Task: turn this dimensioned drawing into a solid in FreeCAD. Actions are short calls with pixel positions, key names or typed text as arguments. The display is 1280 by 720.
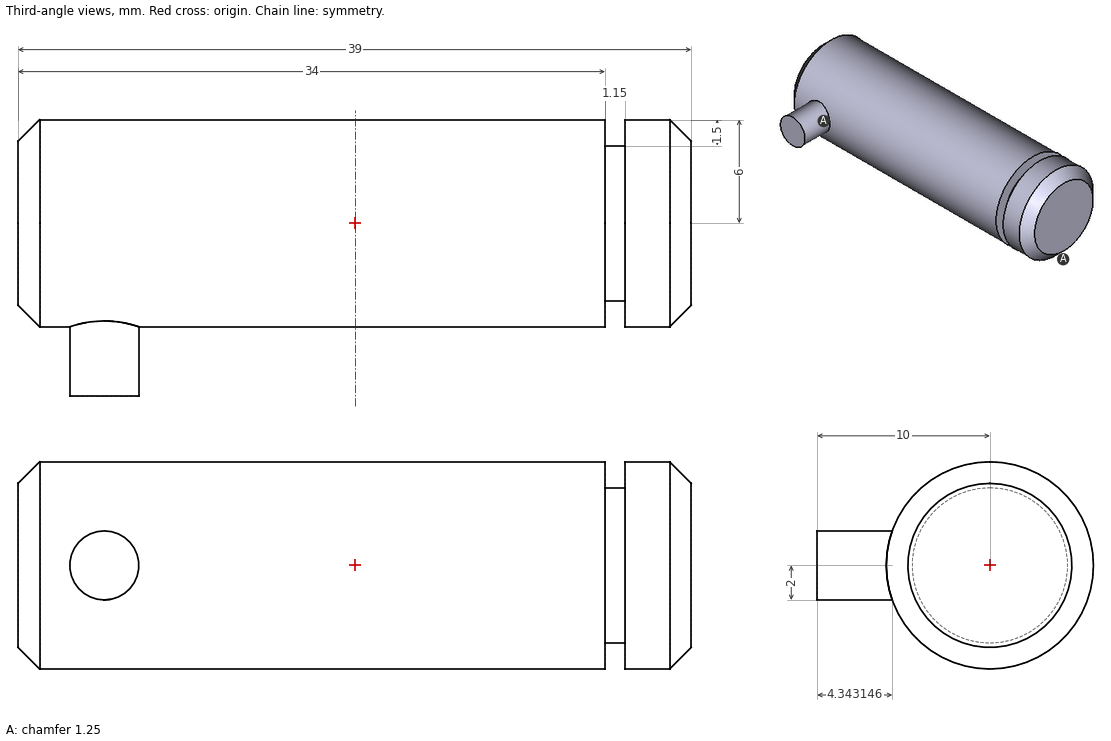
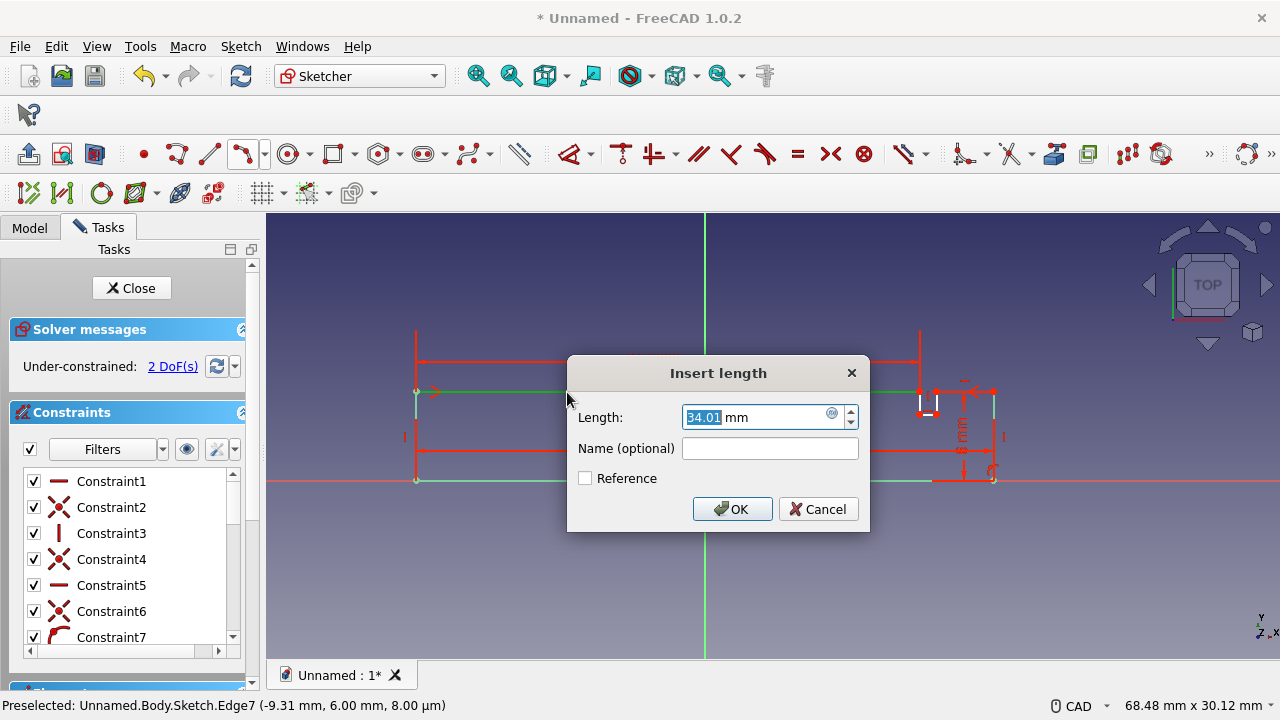
text(34)
key(Return)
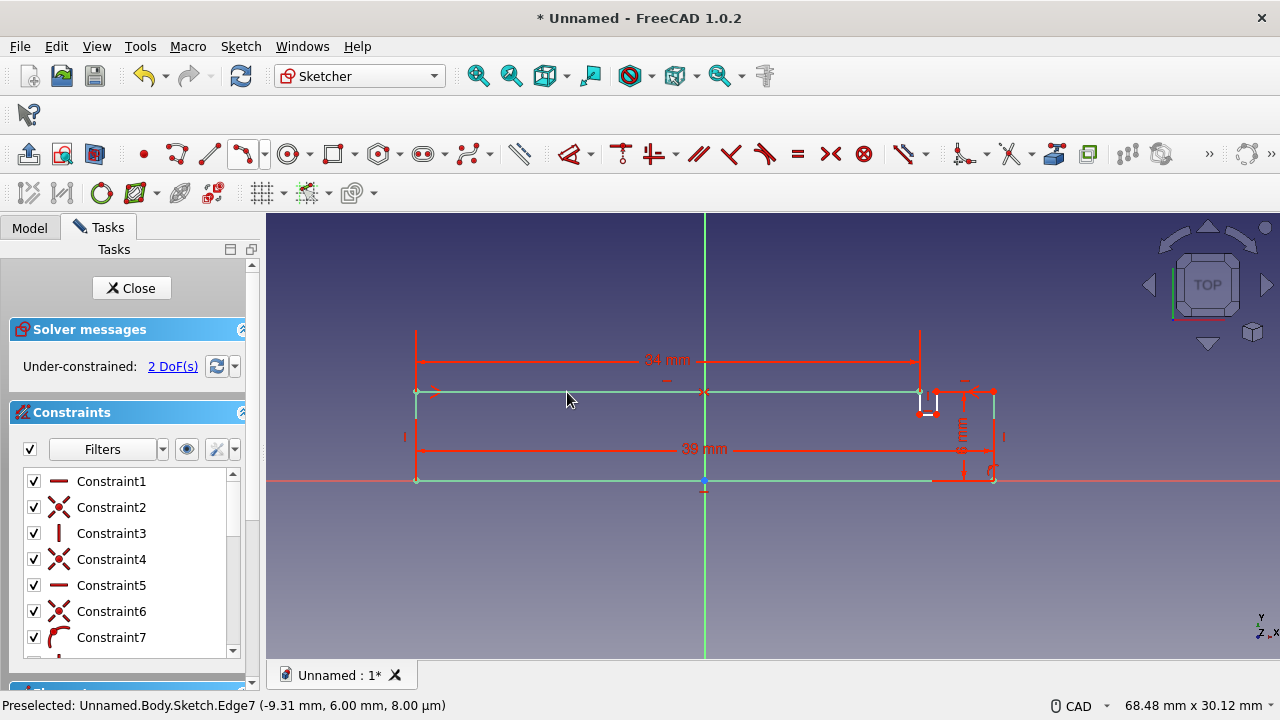
scroll(937, 406, up, 3)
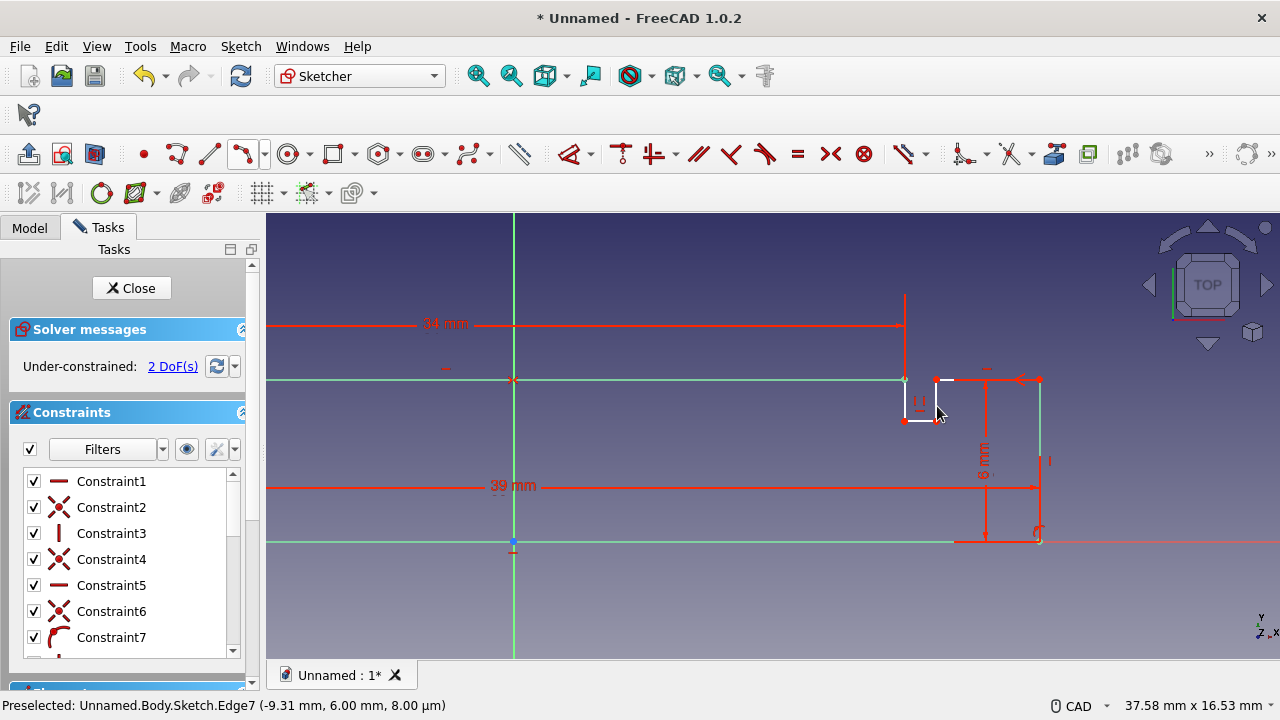
click(936, 405)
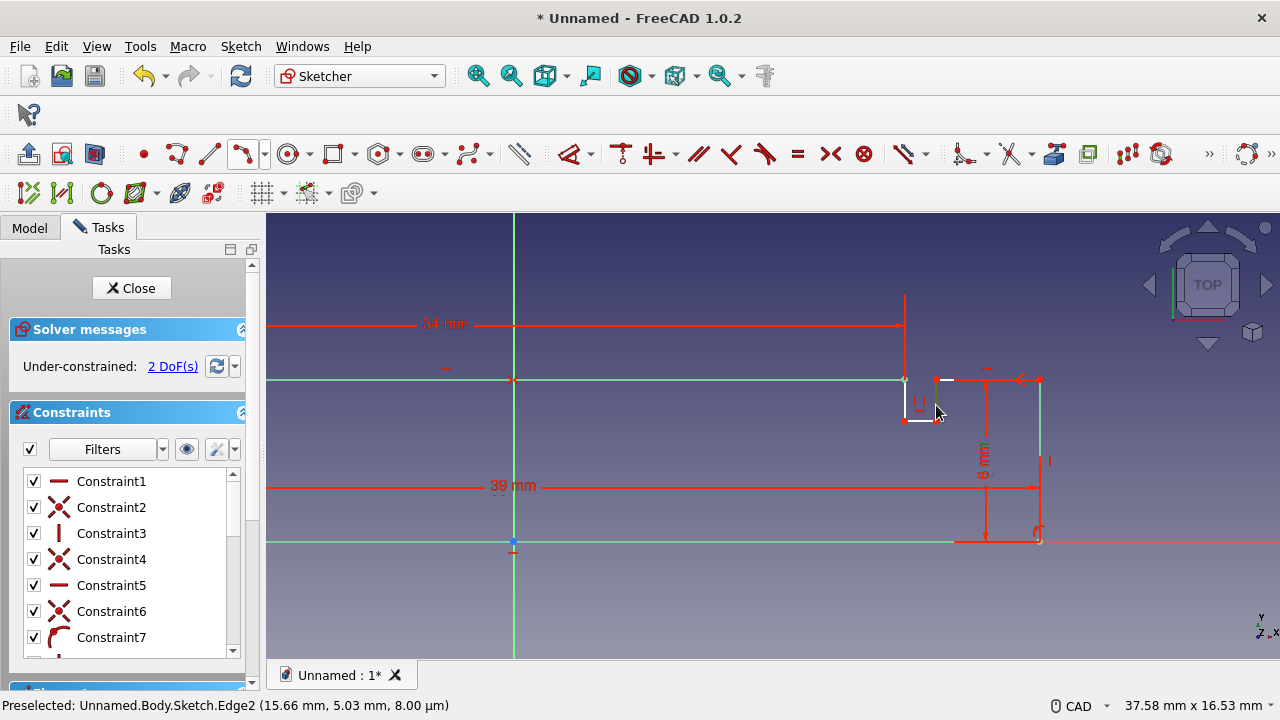
key(i)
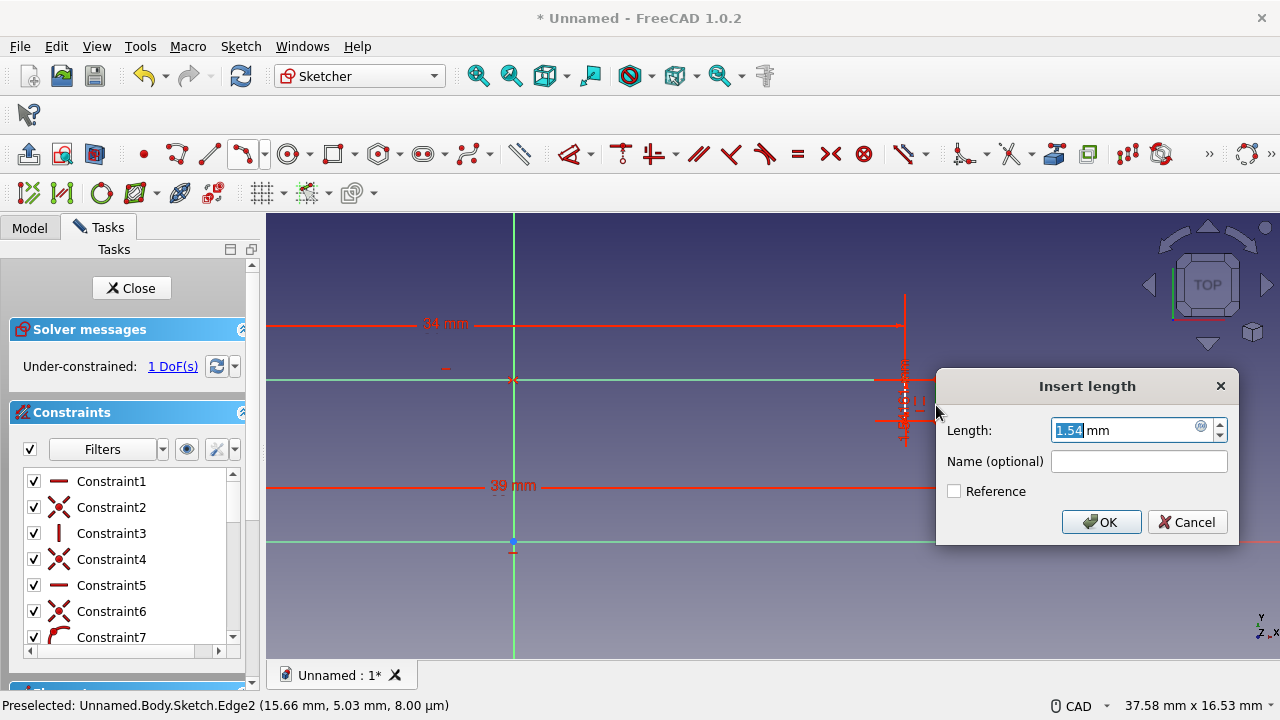
text(1.5)
key(Return)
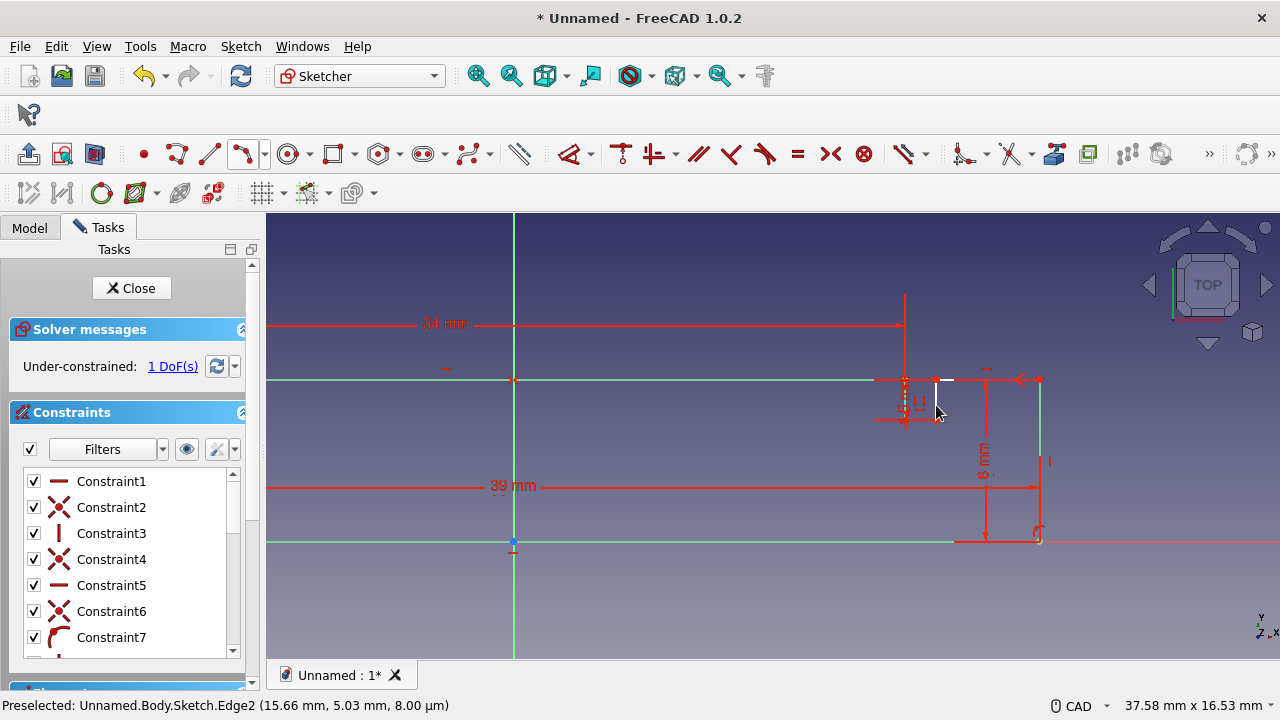
scroll(914, 420, up, 2)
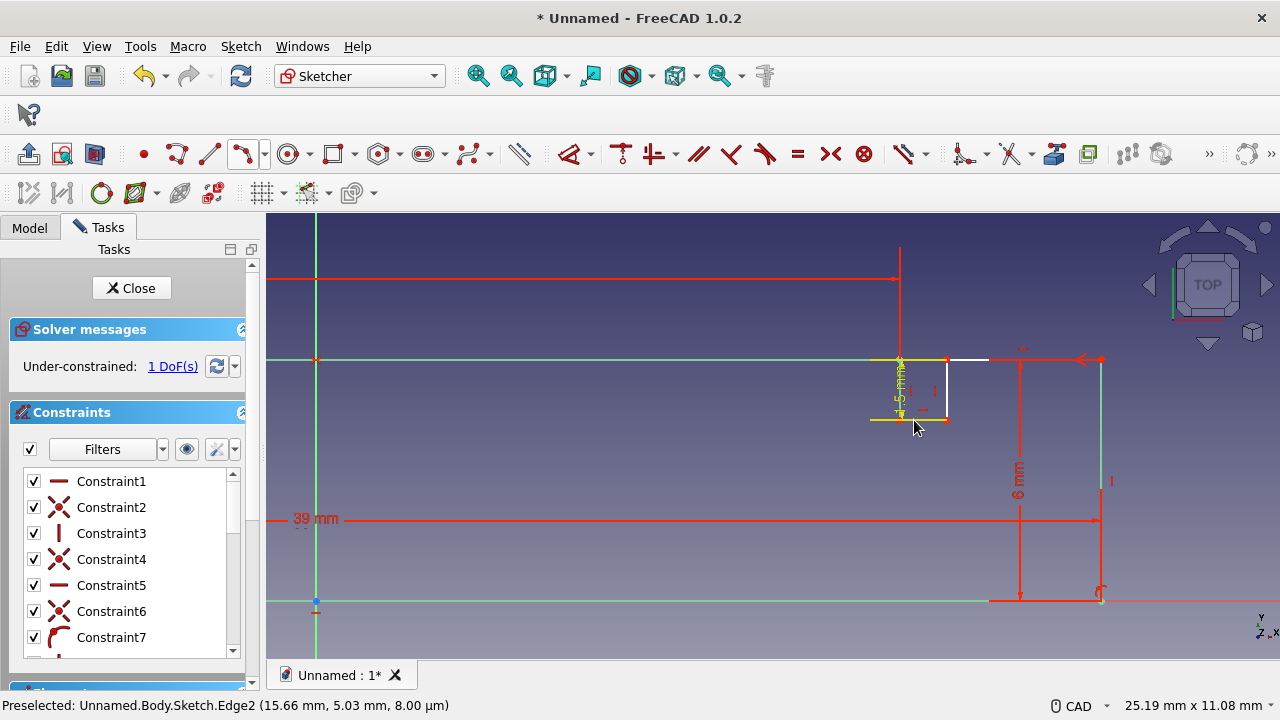
click(914, 420)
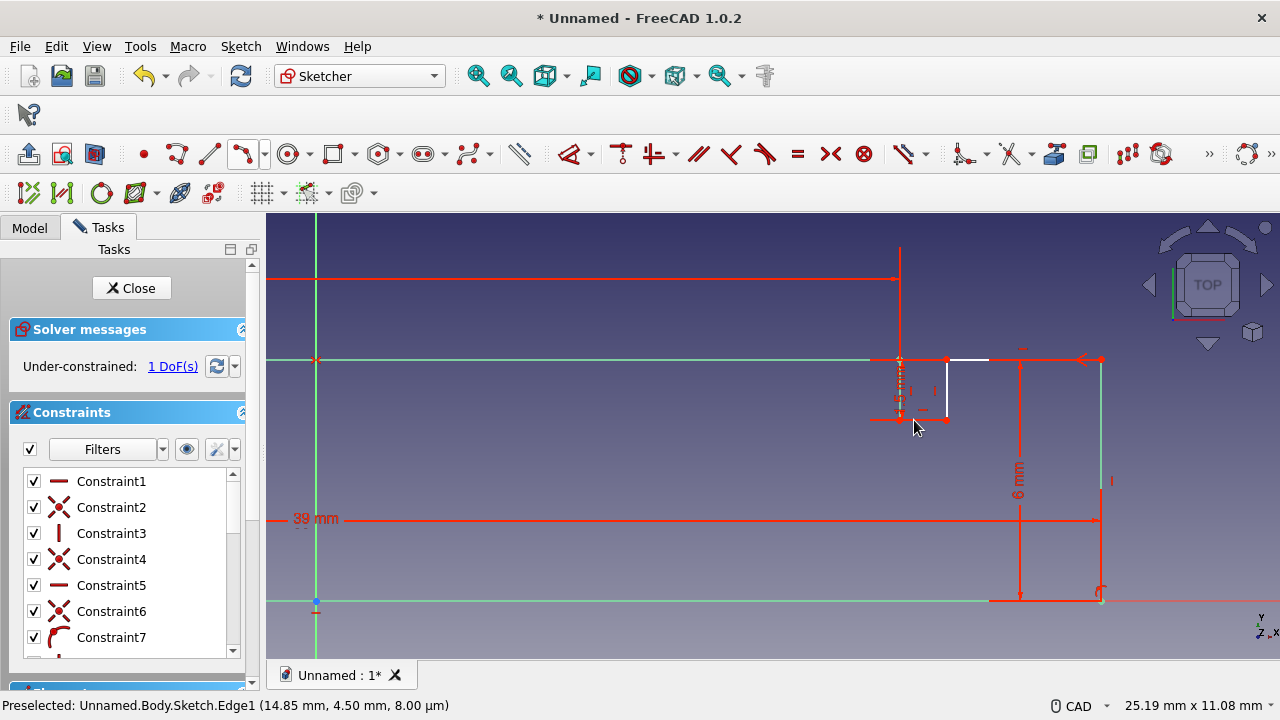
key(l)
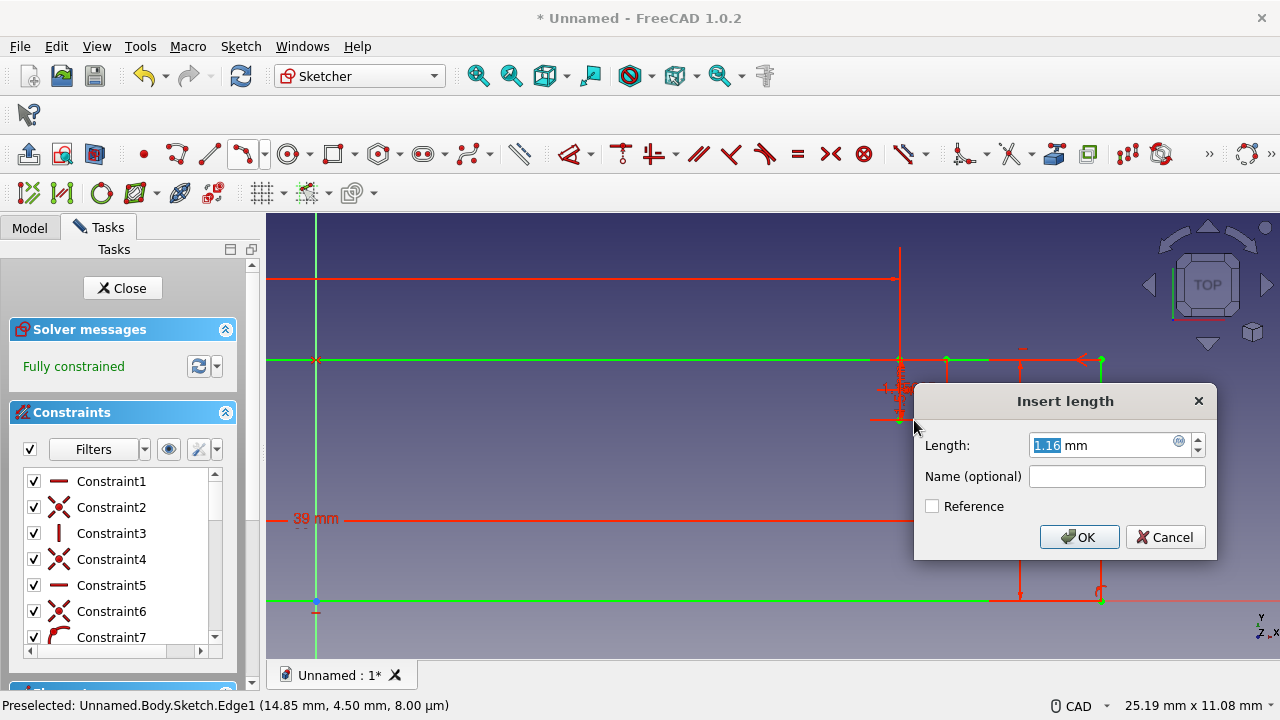
text(1.15)
key(Return)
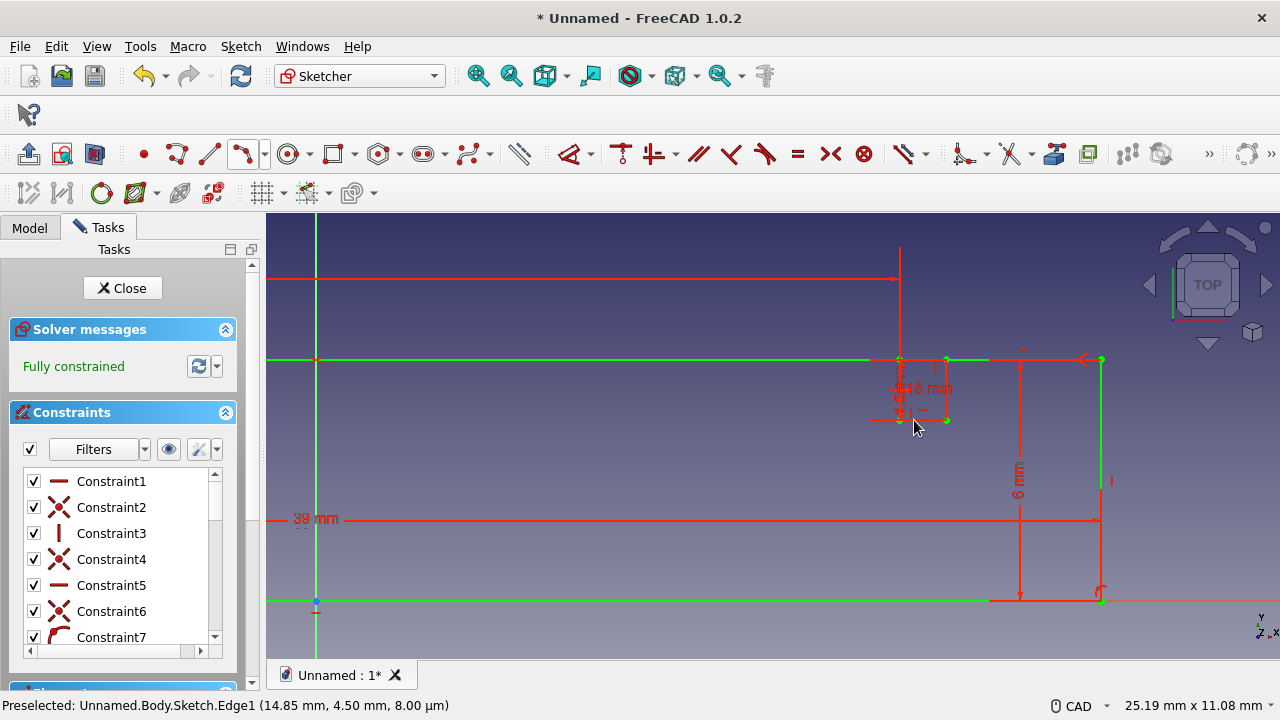
click(123, 288)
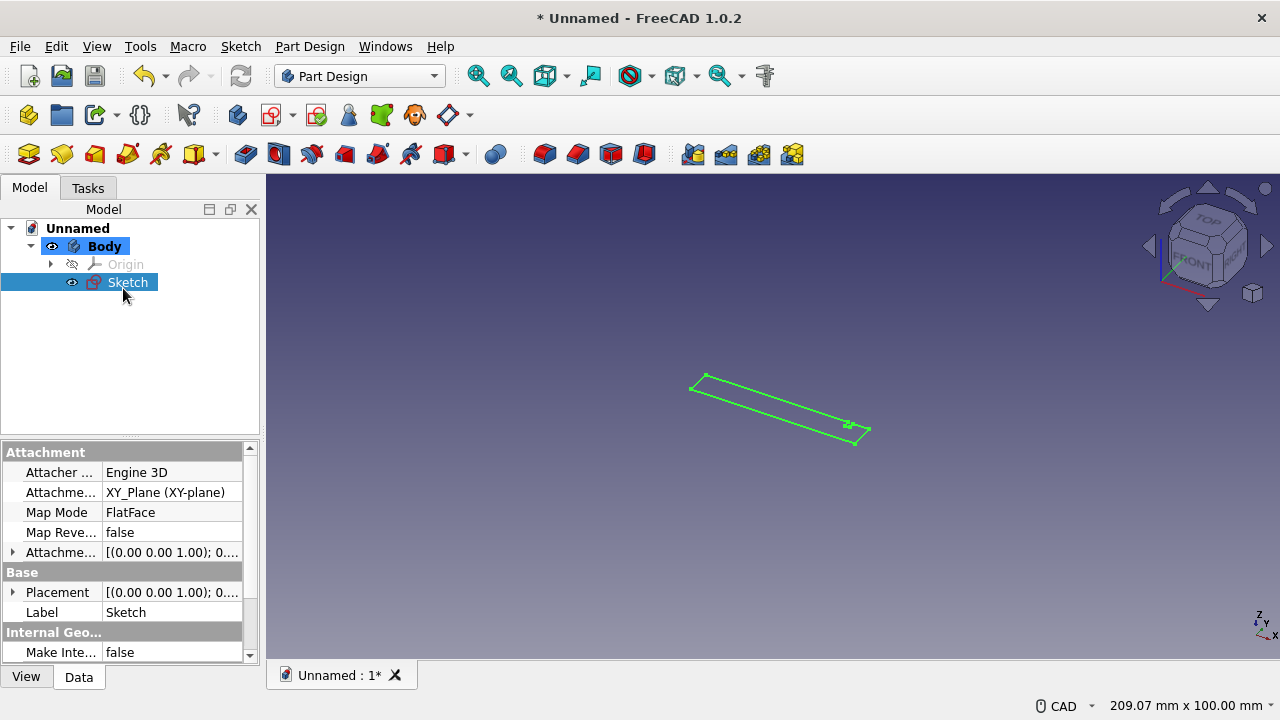
click(62, 154)